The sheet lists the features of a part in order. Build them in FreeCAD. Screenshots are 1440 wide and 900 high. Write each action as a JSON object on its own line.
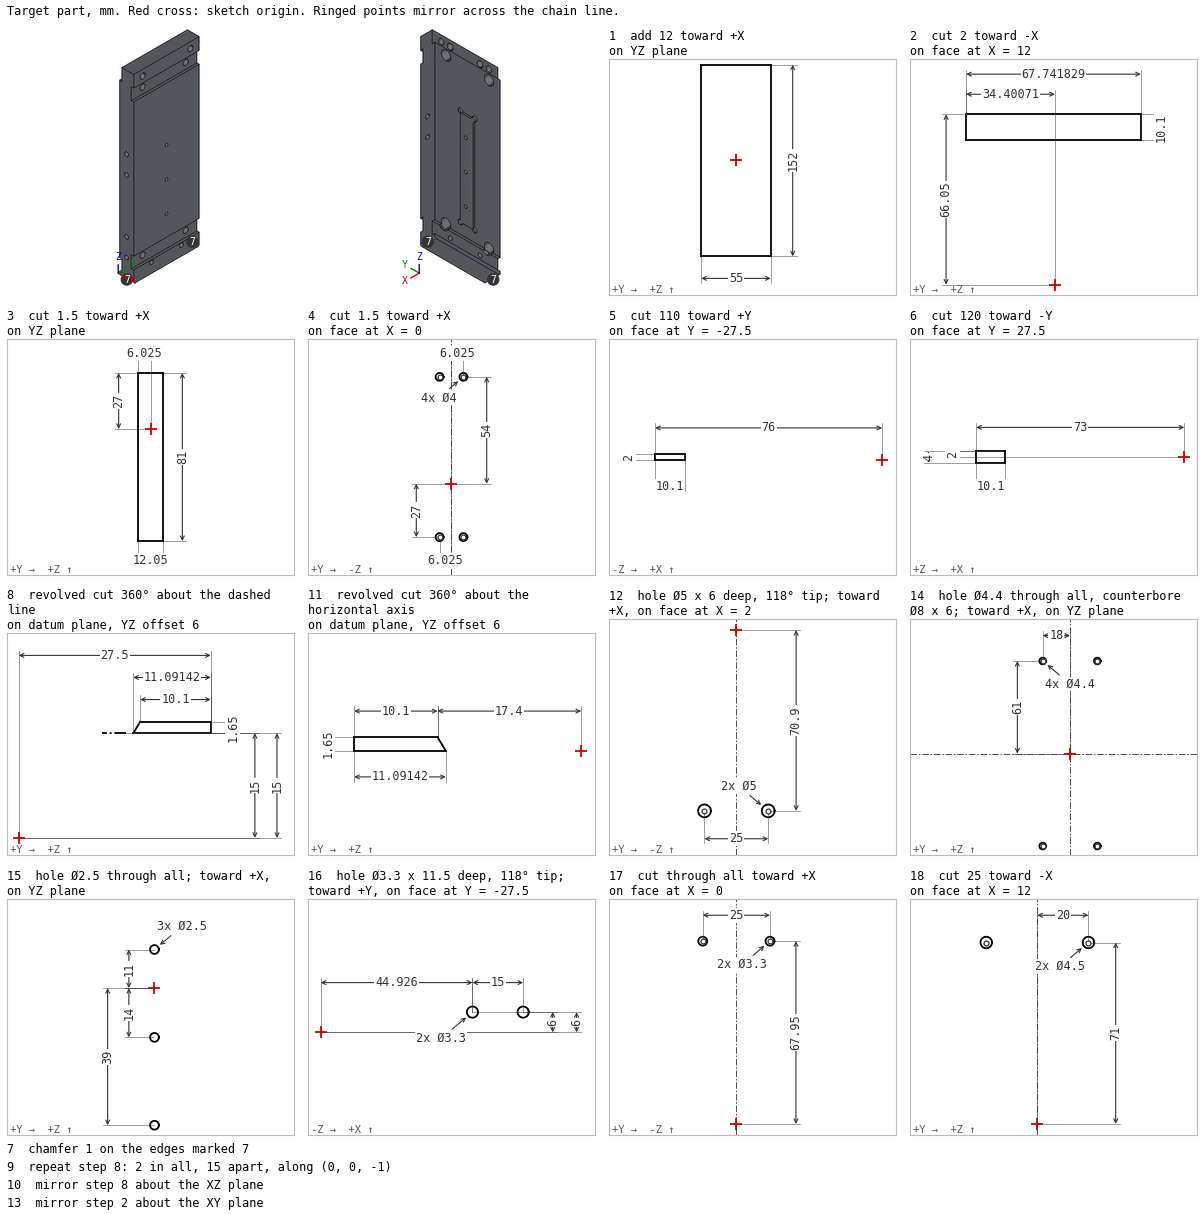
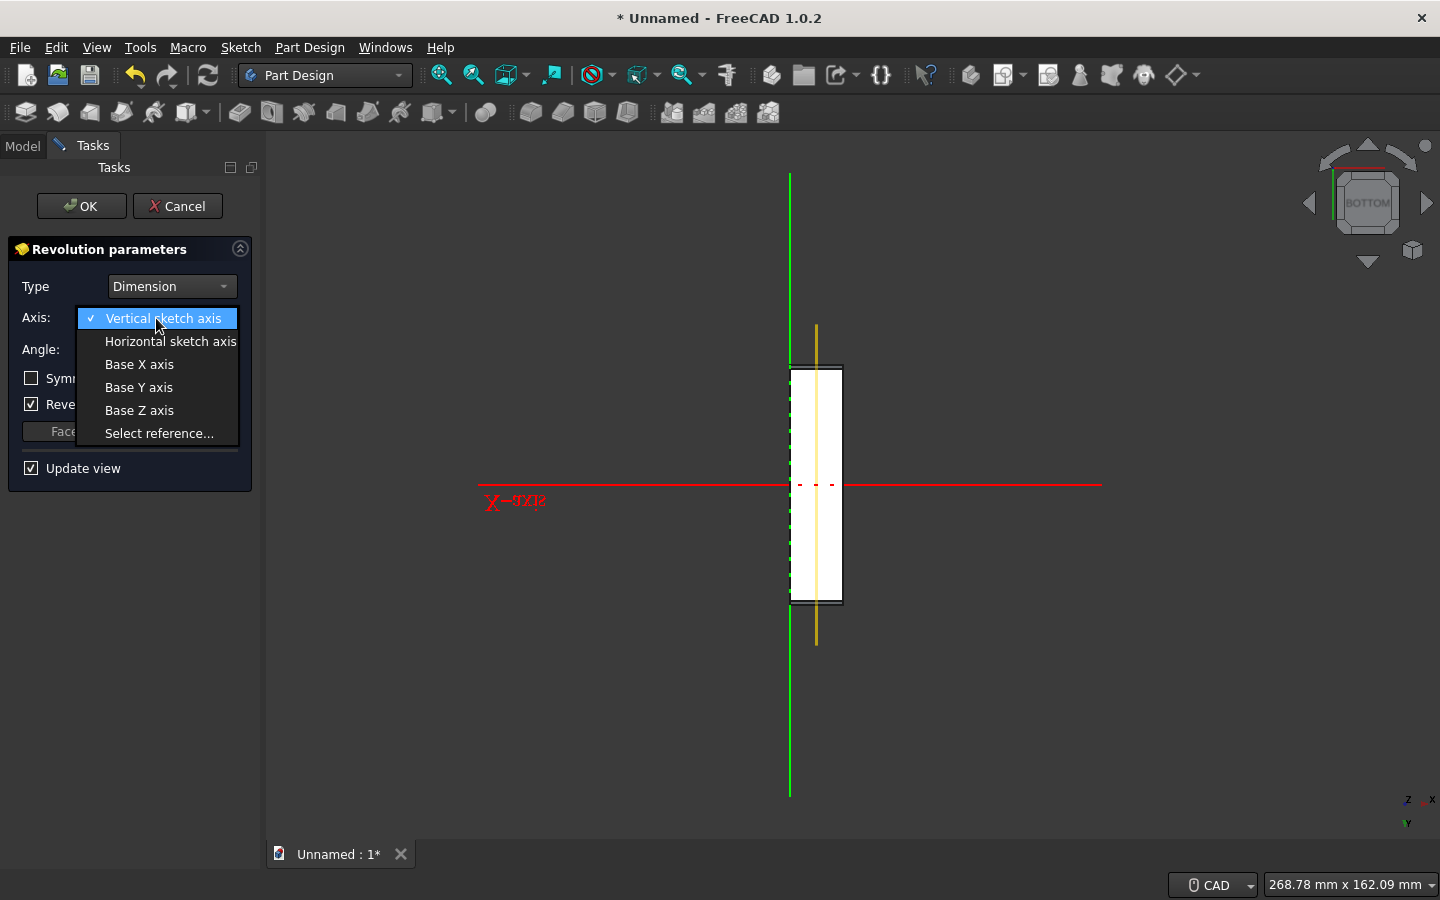
{"action": "left_click", "coordinate": [156, 342]}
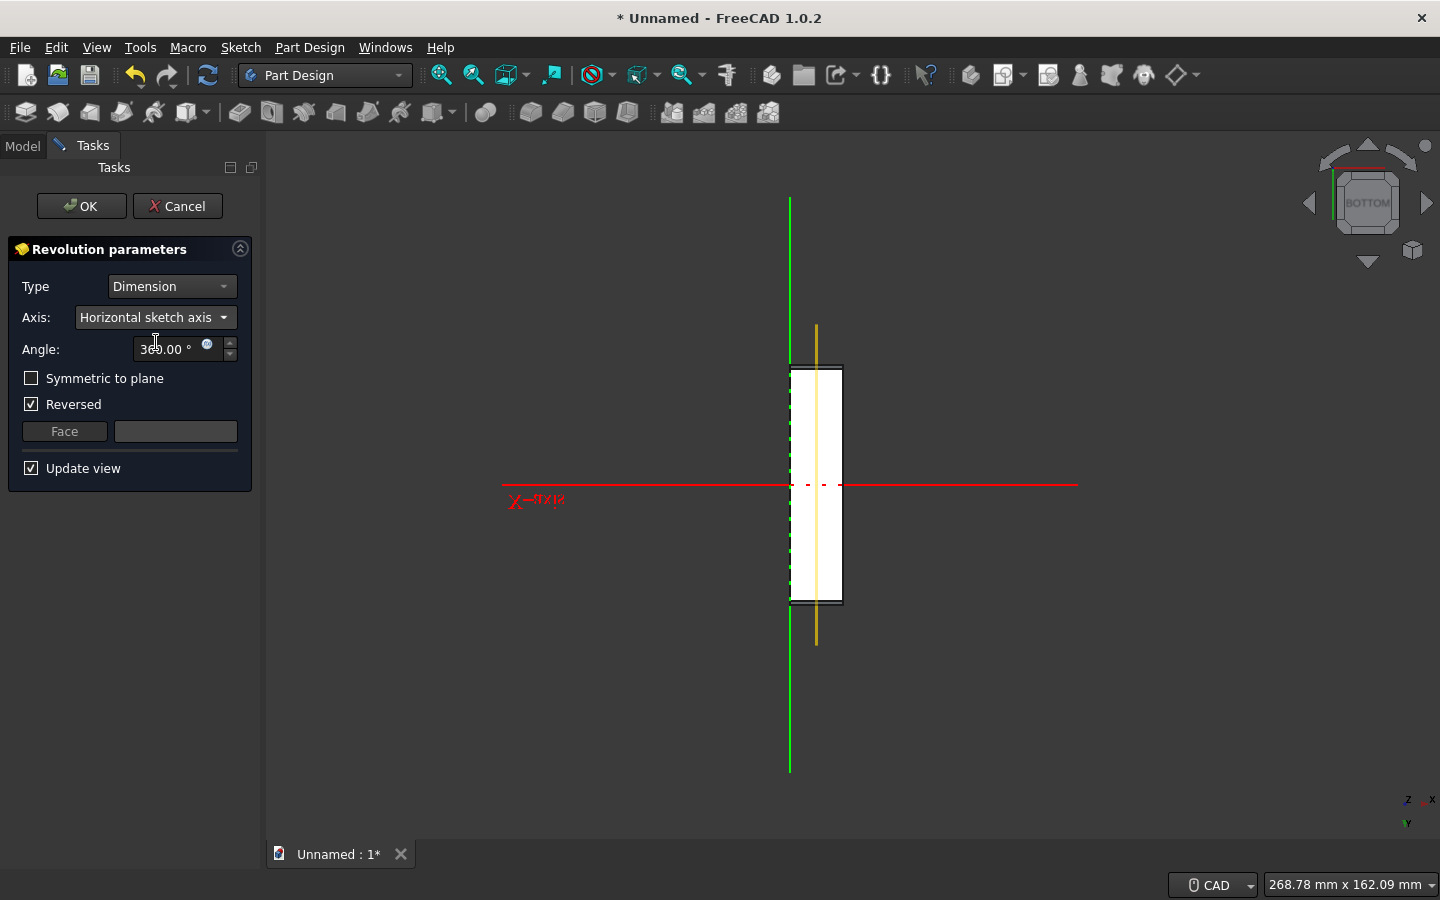
{"action": "left_click", "coordinate": [82, 206]}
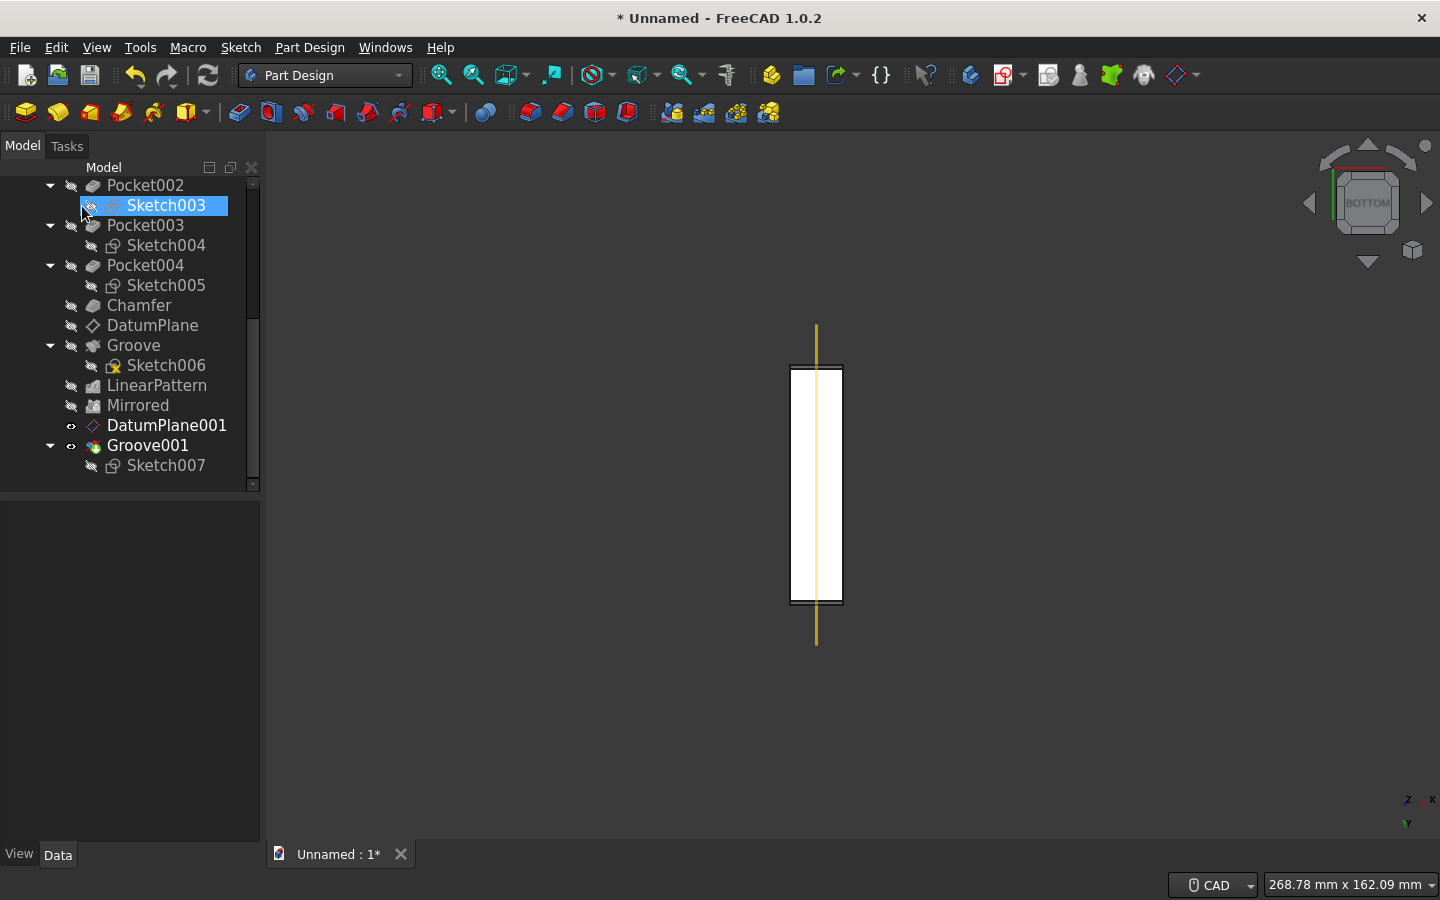
{"action": "left_click", "coordinate": [116, 426]}
{"action": "key", "text": "space"}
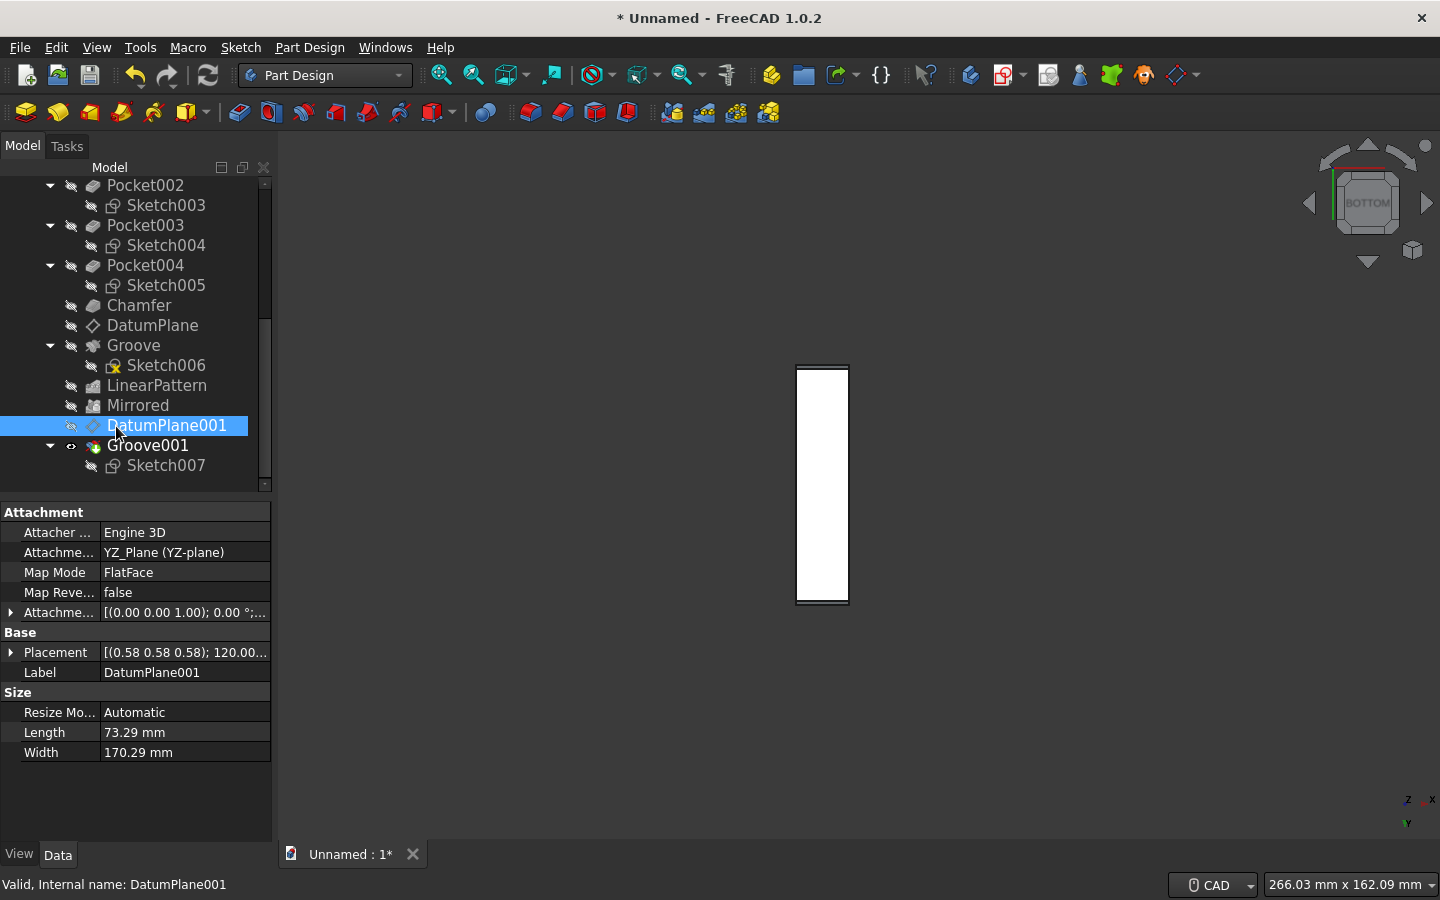
{"action": "left_click", "coordinate": [442, 76]}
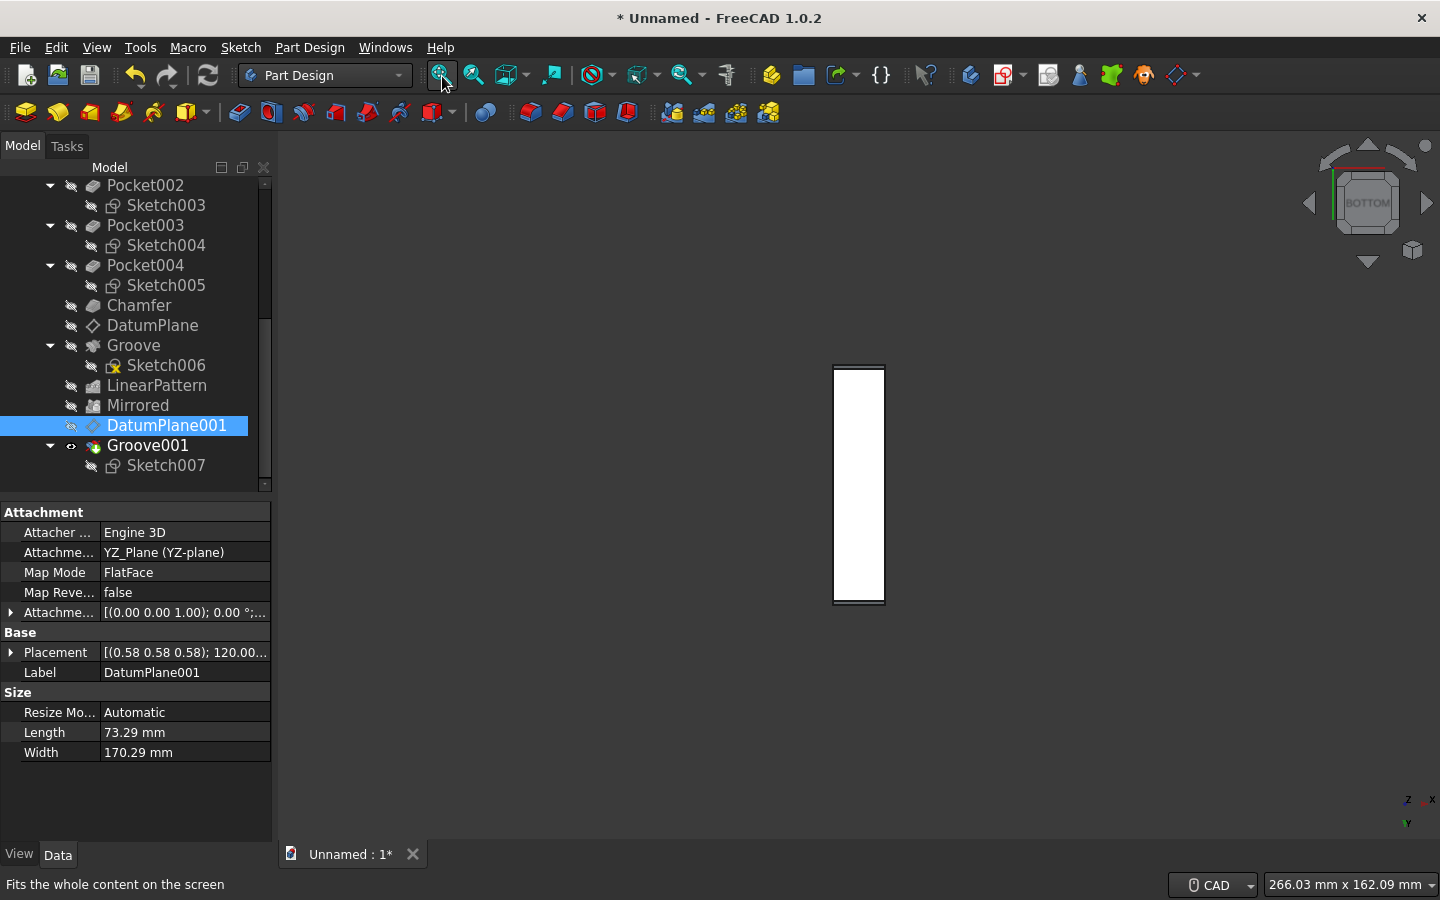
{"action": "key", "text": "6"}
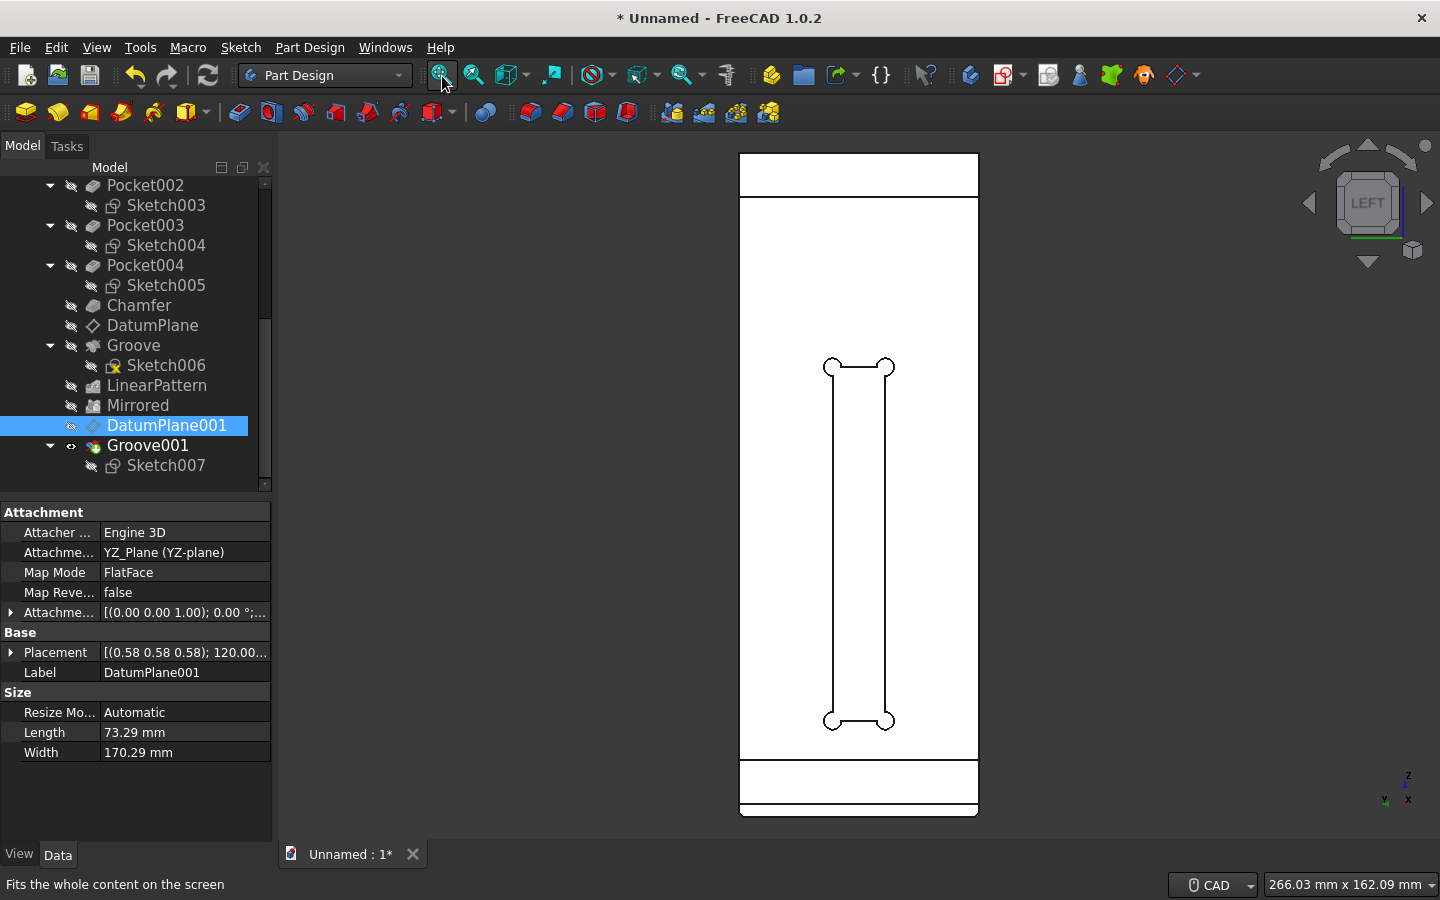
{"action": "left_click", "coordinate": [790, 781]}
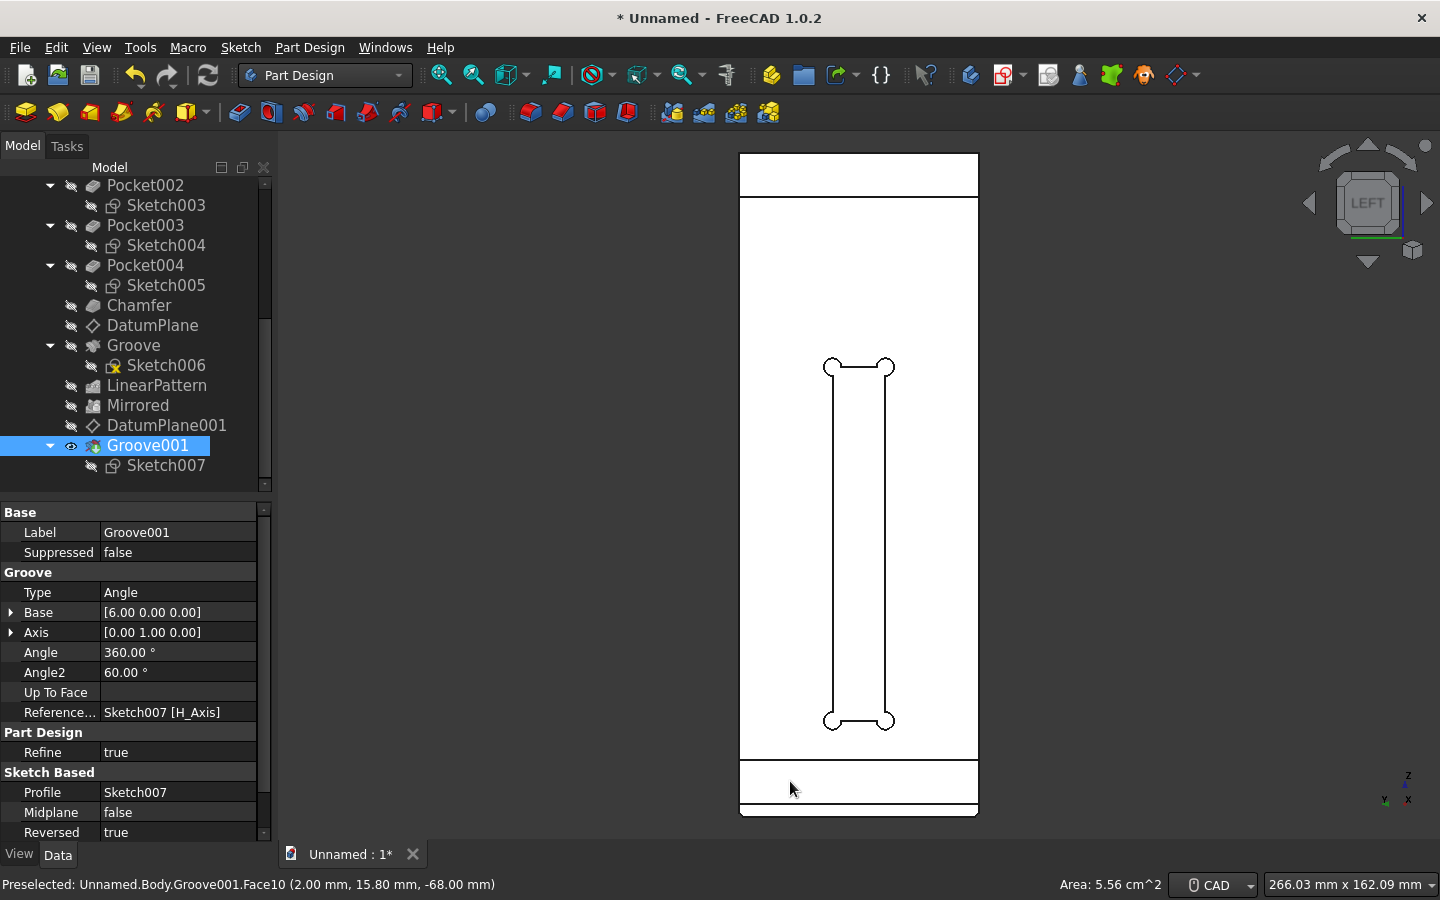
{"action": "left_click", "coordinate": [1004, 76]}